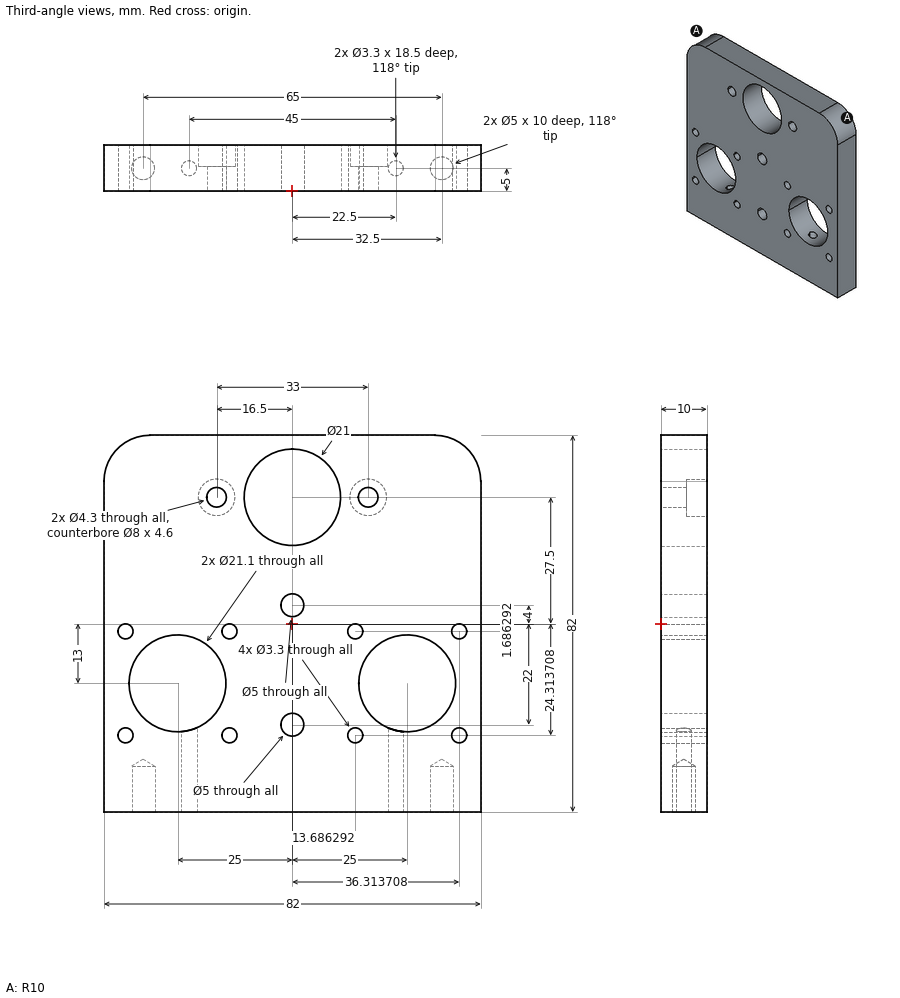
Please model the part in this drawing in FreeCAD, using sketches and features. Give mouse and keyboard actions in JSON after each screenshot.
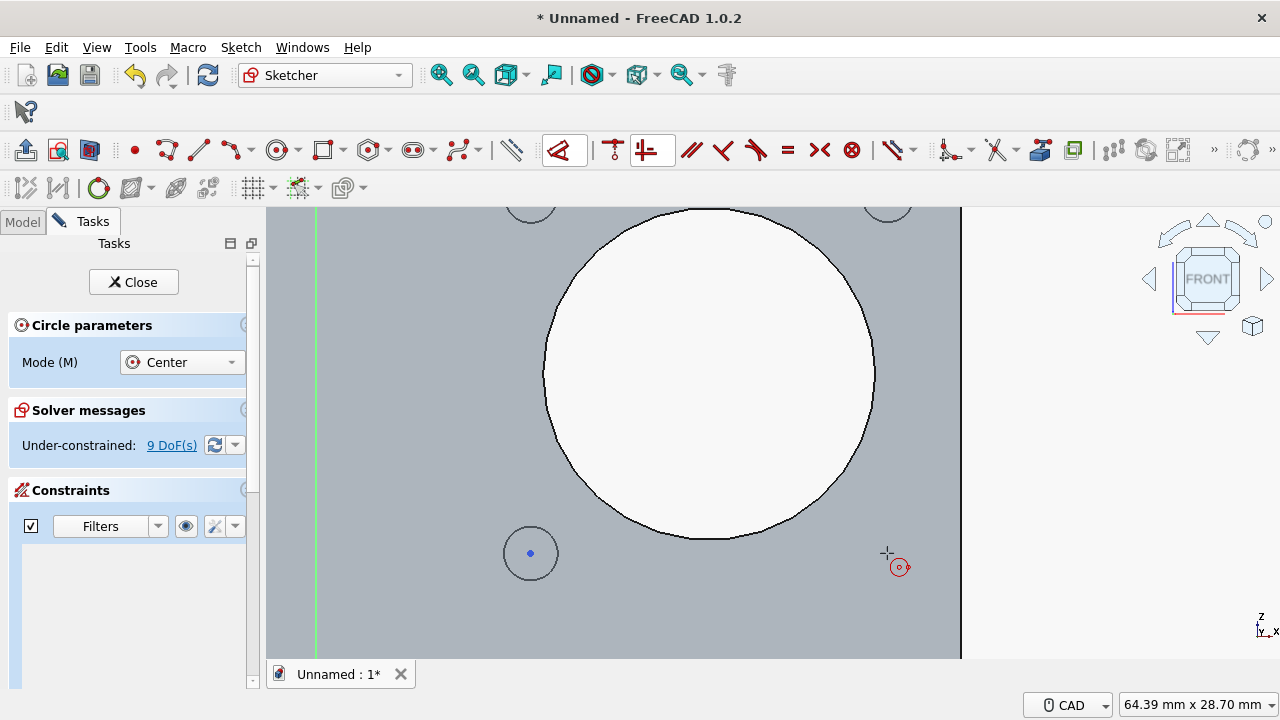
{"action": "left_click", "coordinate": [887, 552]}
{"action": "left_click", "coordinate": [906, 534]}
{"action": "key", "text": "Escape"}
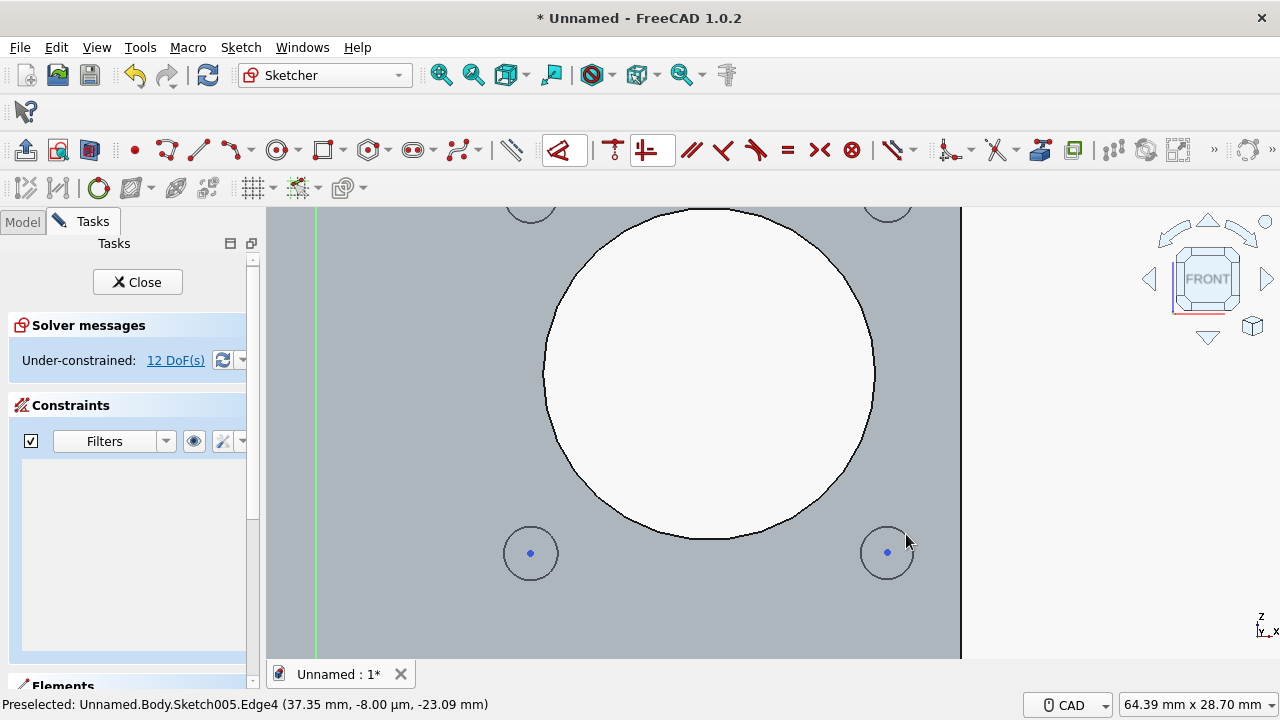
{"action": "left_click", "coordinate": [550, 534]}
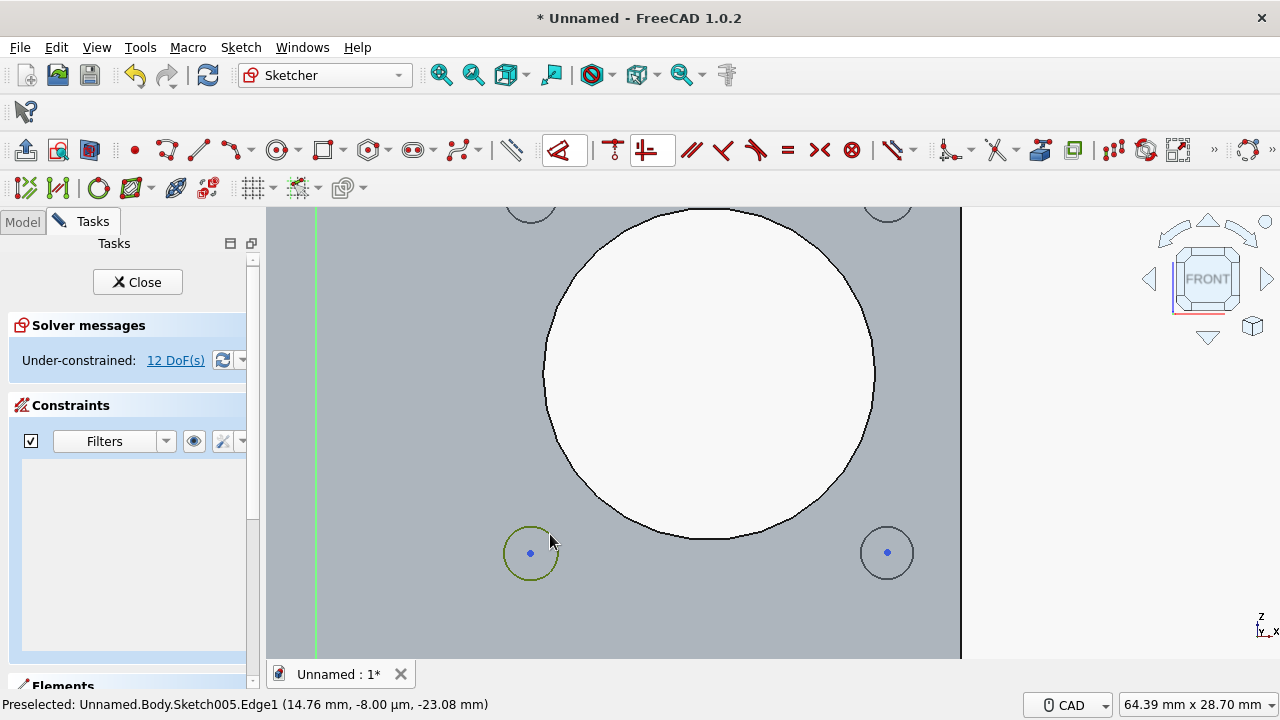
{"action": "scroll", "coordinate": [888, 554], "scroll_direction": "down", "scroll_amount": 2}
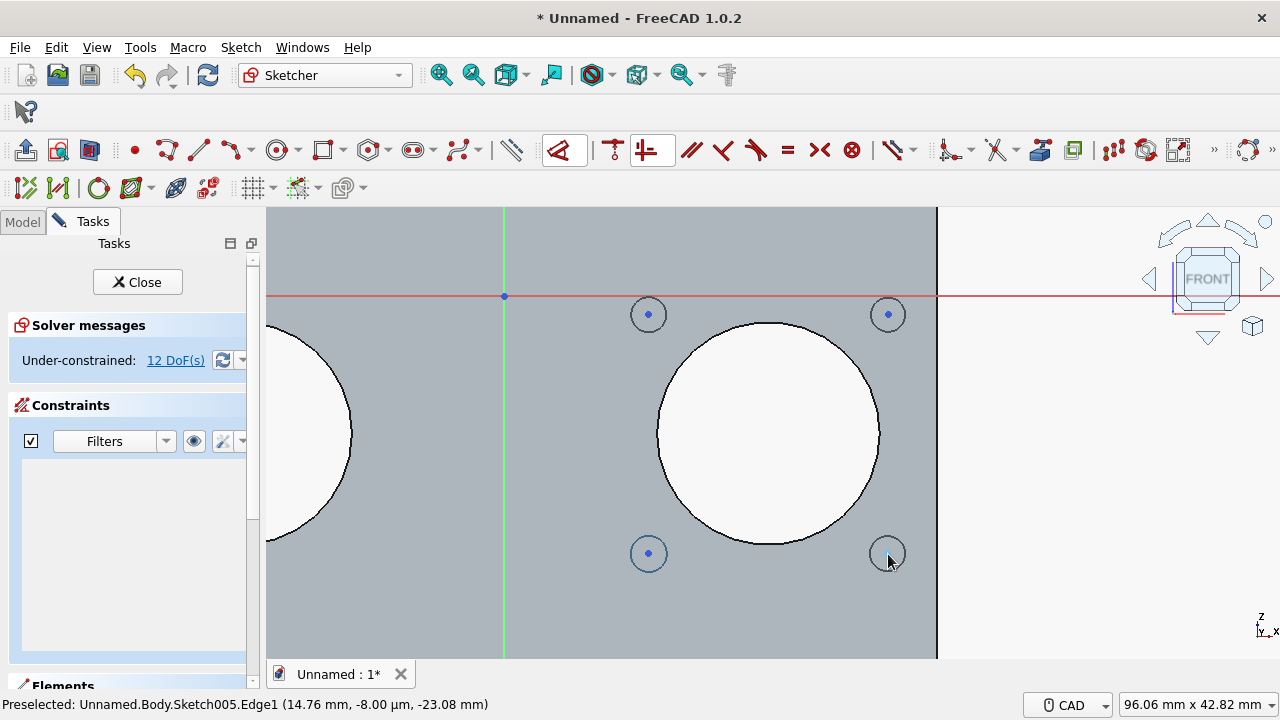
{"action": "left_click", "coordinate": [636, 327]}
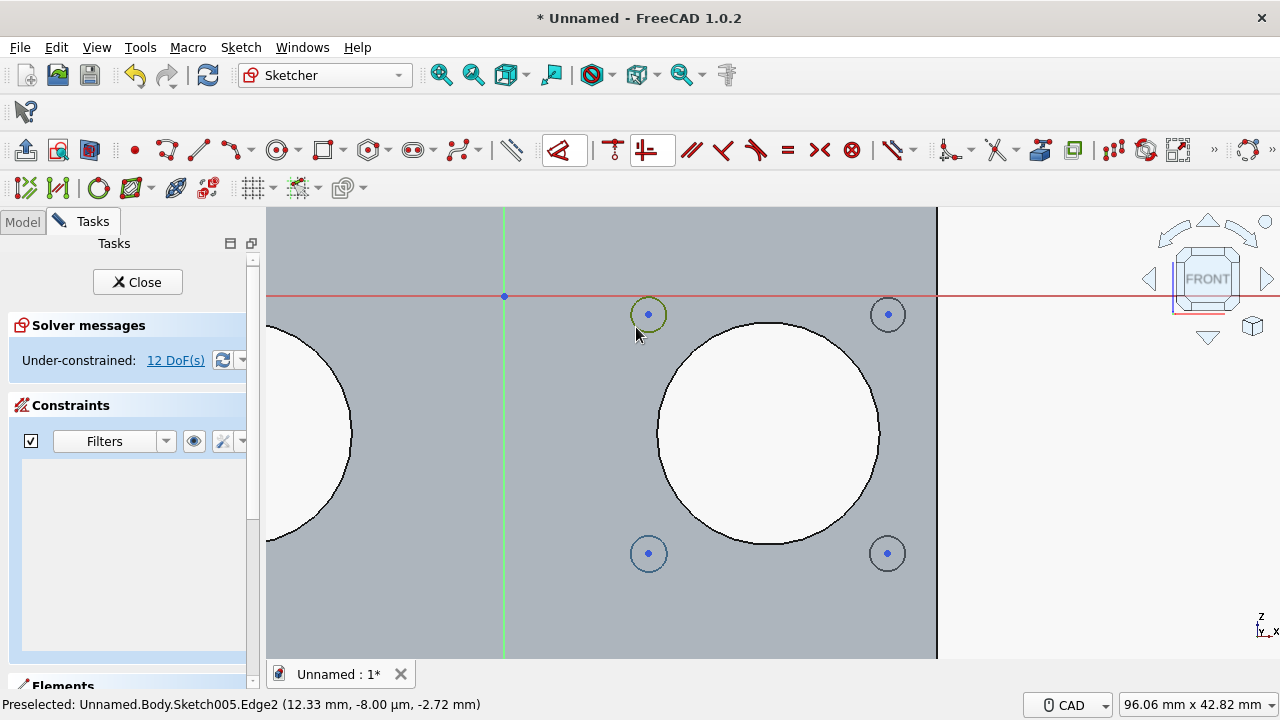
{"action": "left_click", "coordinate": [876, 327]}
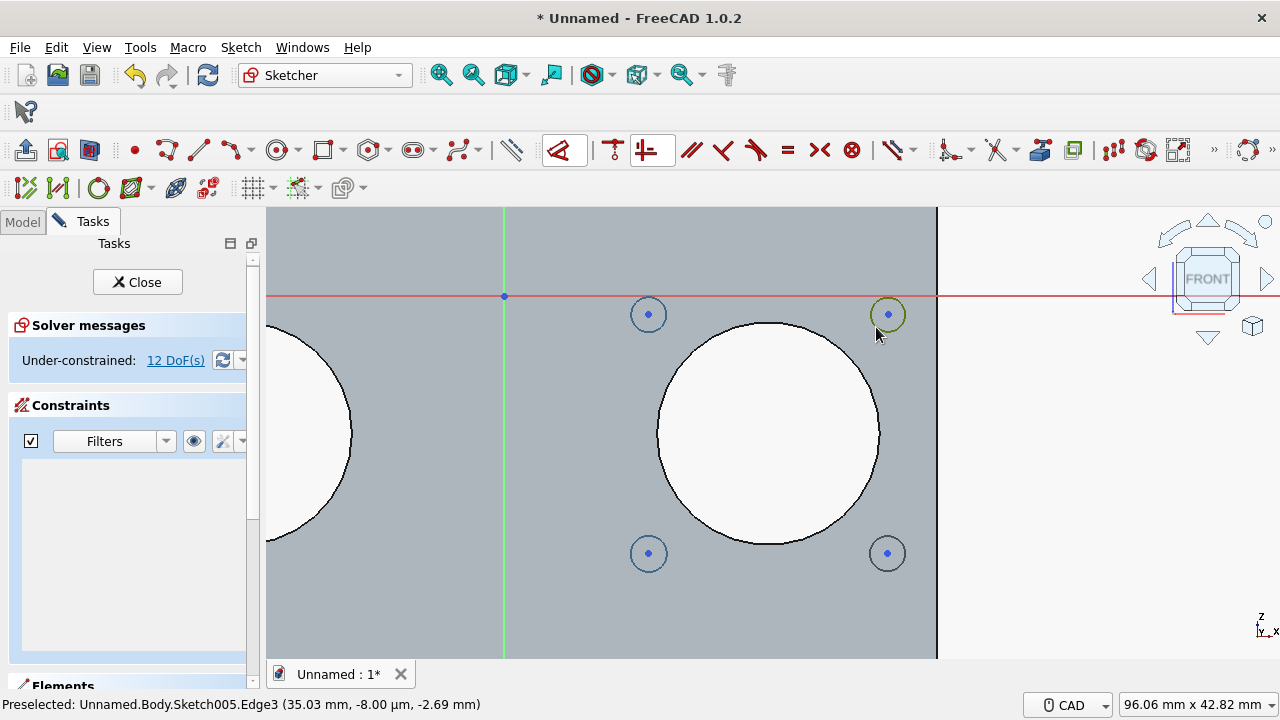
{"action": "left_click", "coordinate": [900, 541]}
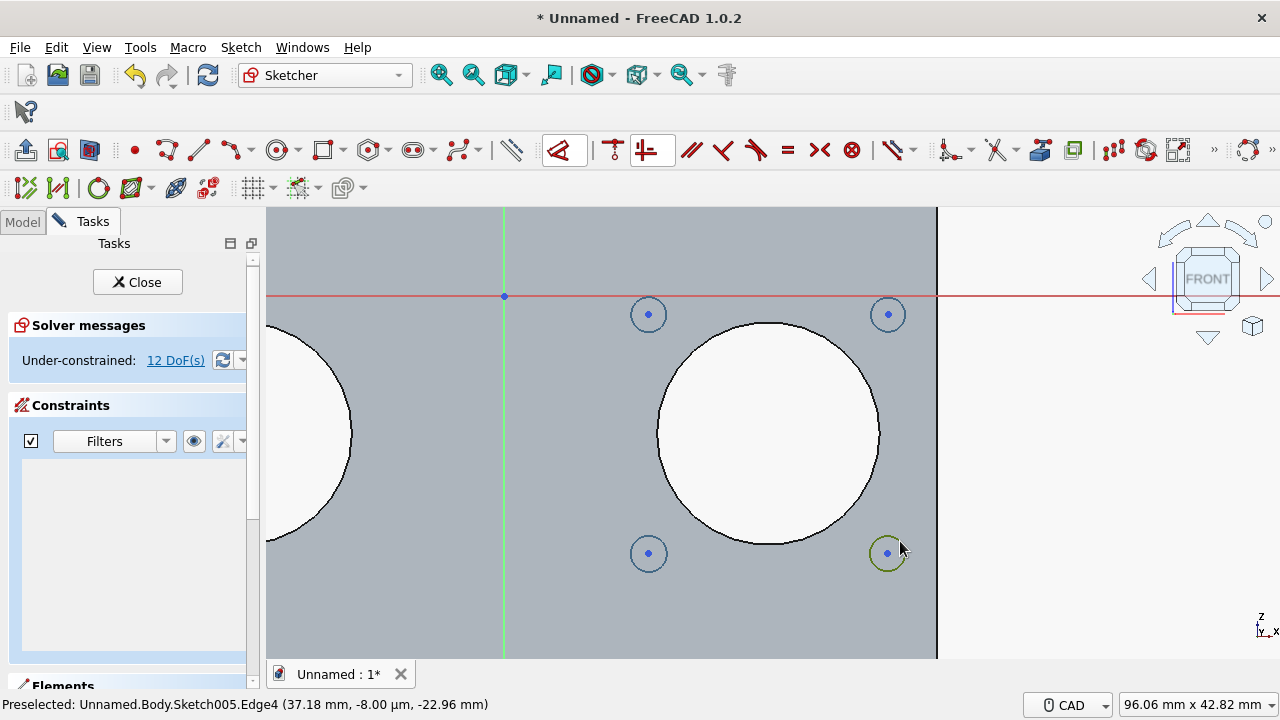
{"action": "left_click", "coordinate": [788, 150]}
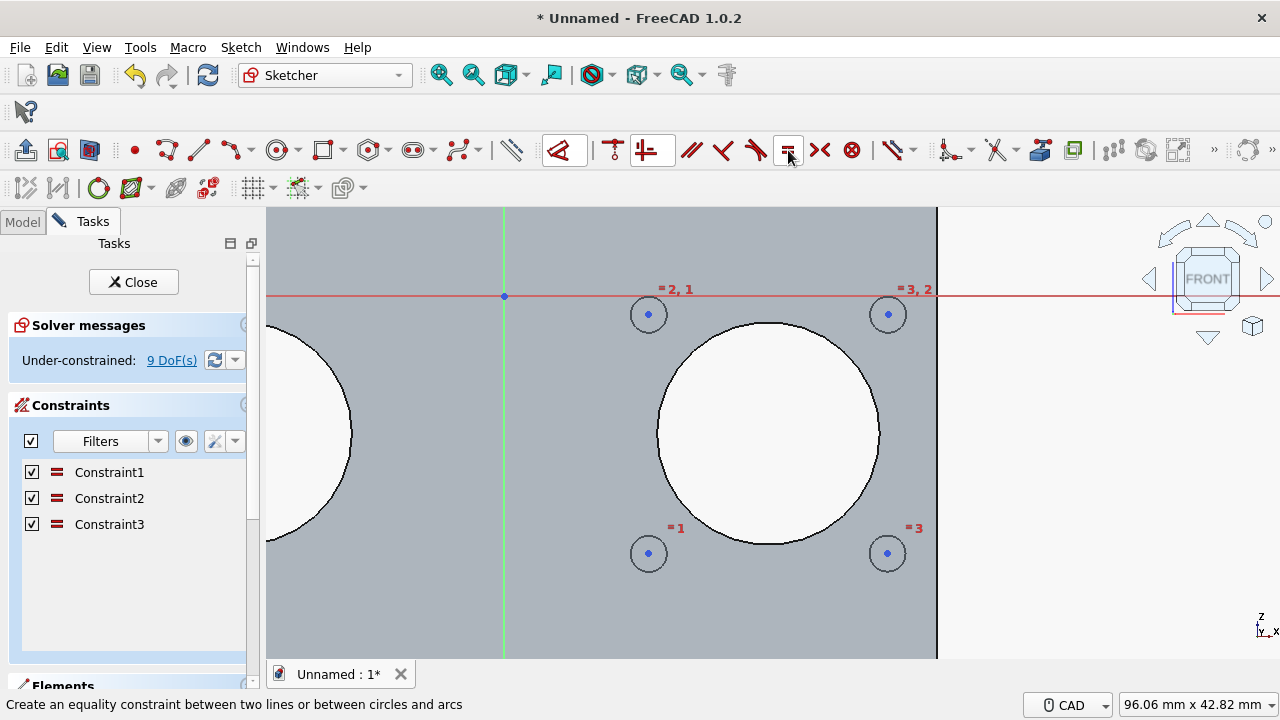
{"action": "left_click", "coordinate": [661, 541]}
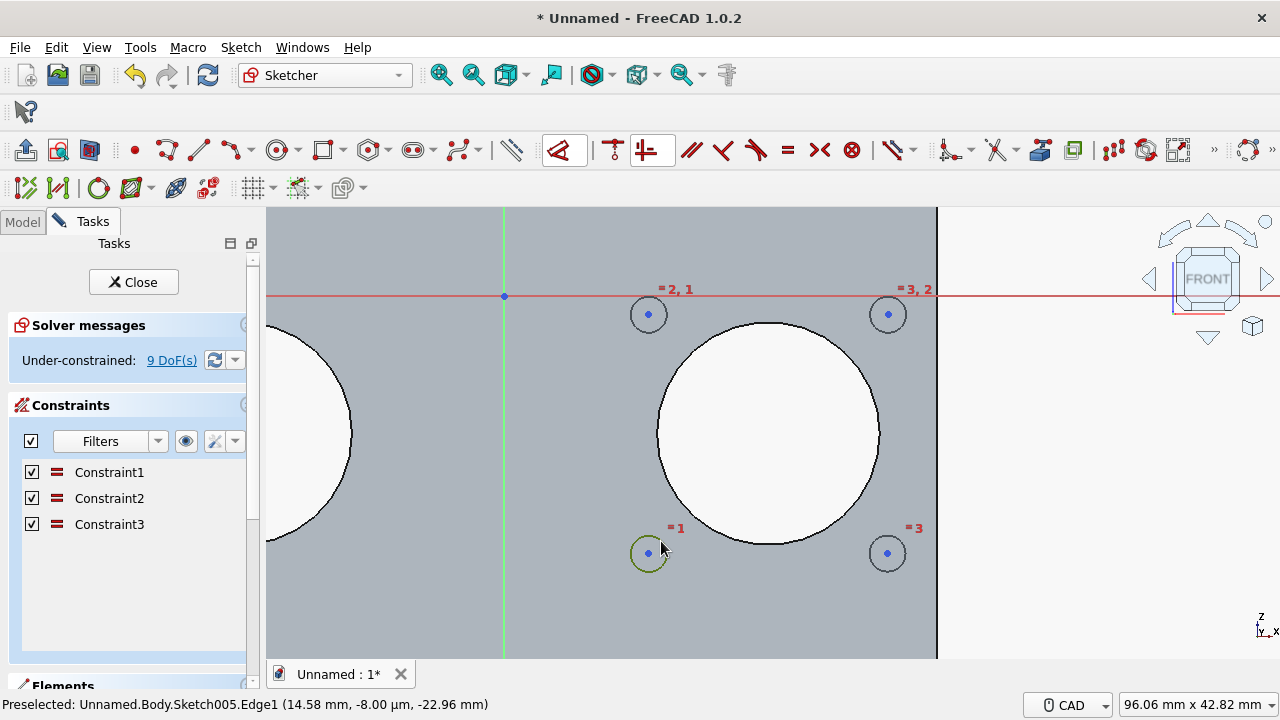
{"action": "key", "text": "k o"}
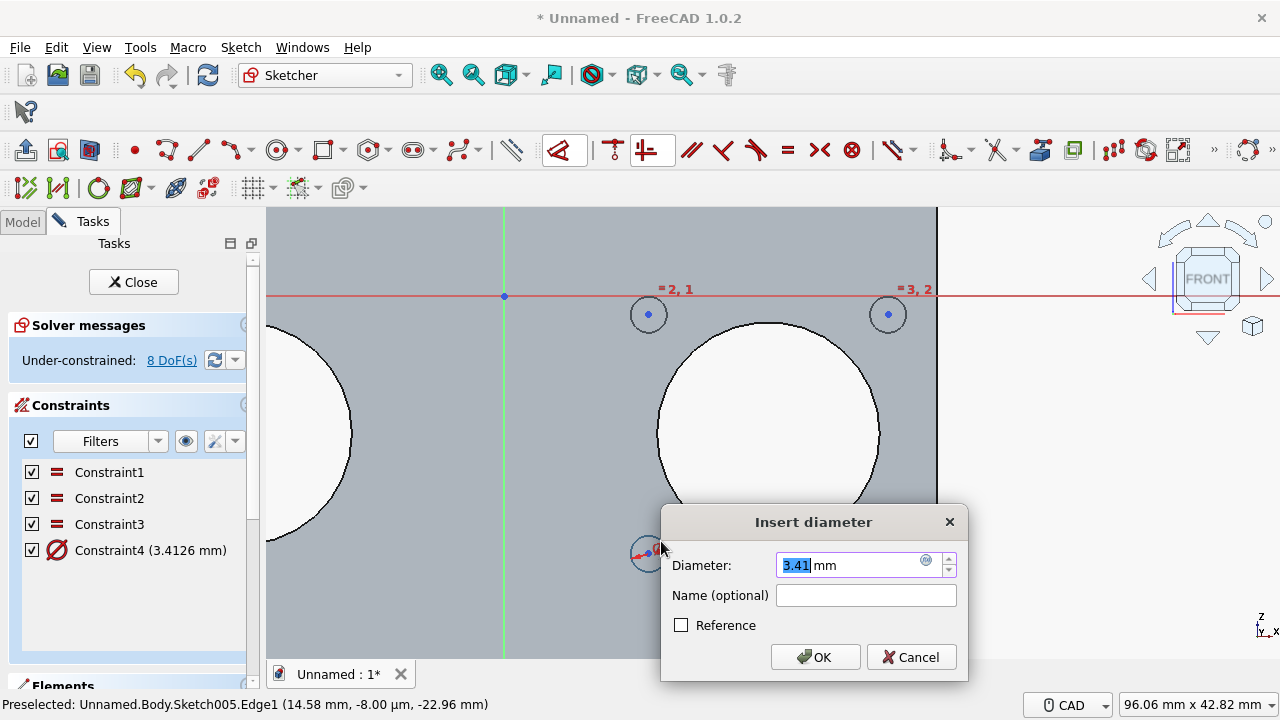
{"action": "type", "text": "3.3"}
{"action": "key", "text": "Return"}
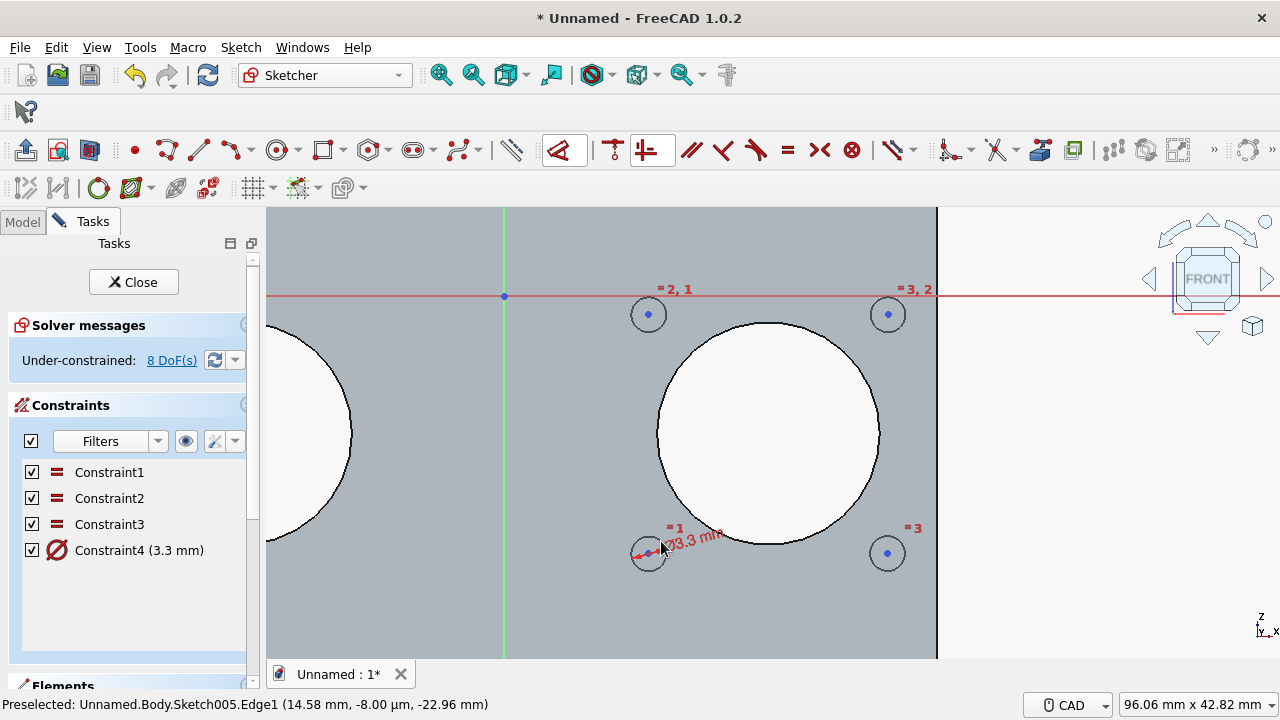
{"action": "scroll", "coordinate": [649, 315], "scroll_direction": "up", "scroll_amount": 5}